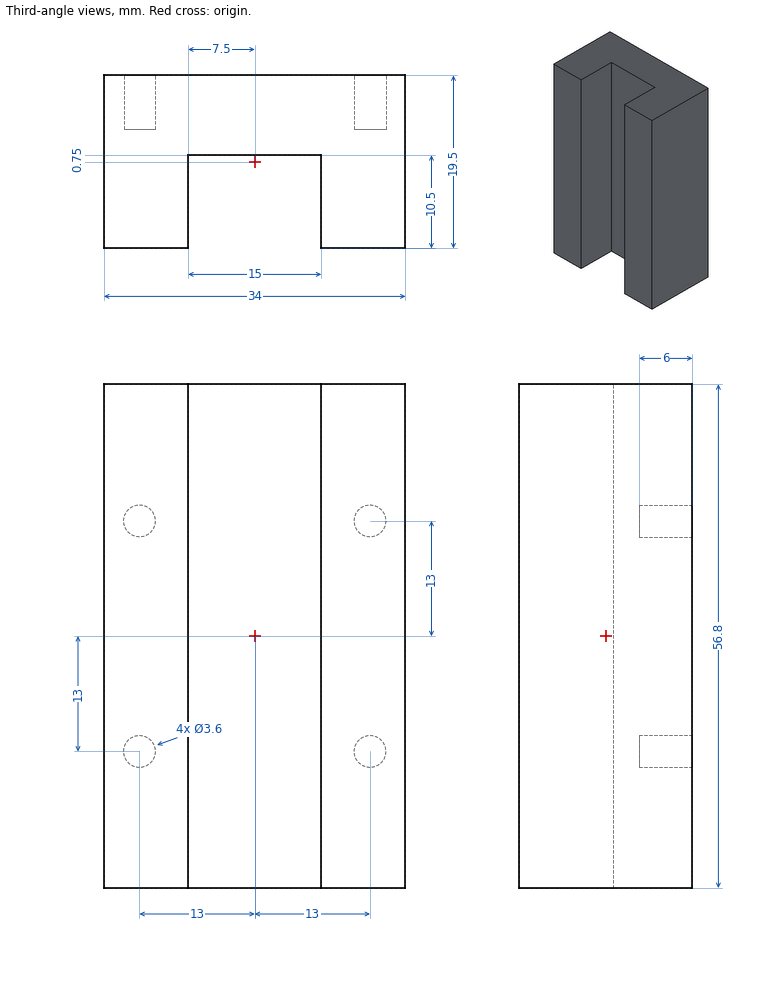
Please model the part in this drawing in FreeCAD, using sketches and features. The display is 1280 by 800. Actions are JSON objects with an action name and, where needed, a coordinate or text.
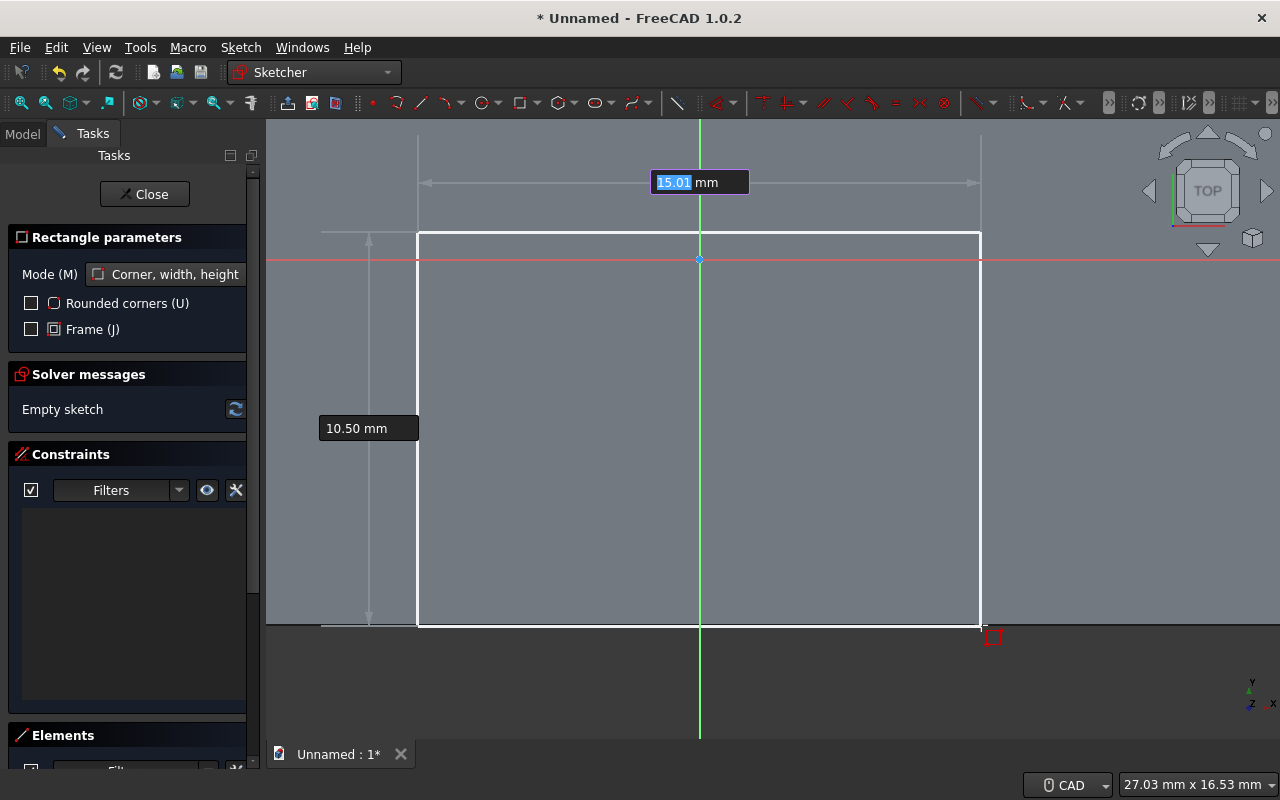
{"action": "type", "text": "15"}
{"action": "key", "text": "Tab"}
{"action": "type", "text": "10.5"}
{"action": "key", "text": "Return"}
{"action": "key", "text": "Escape"}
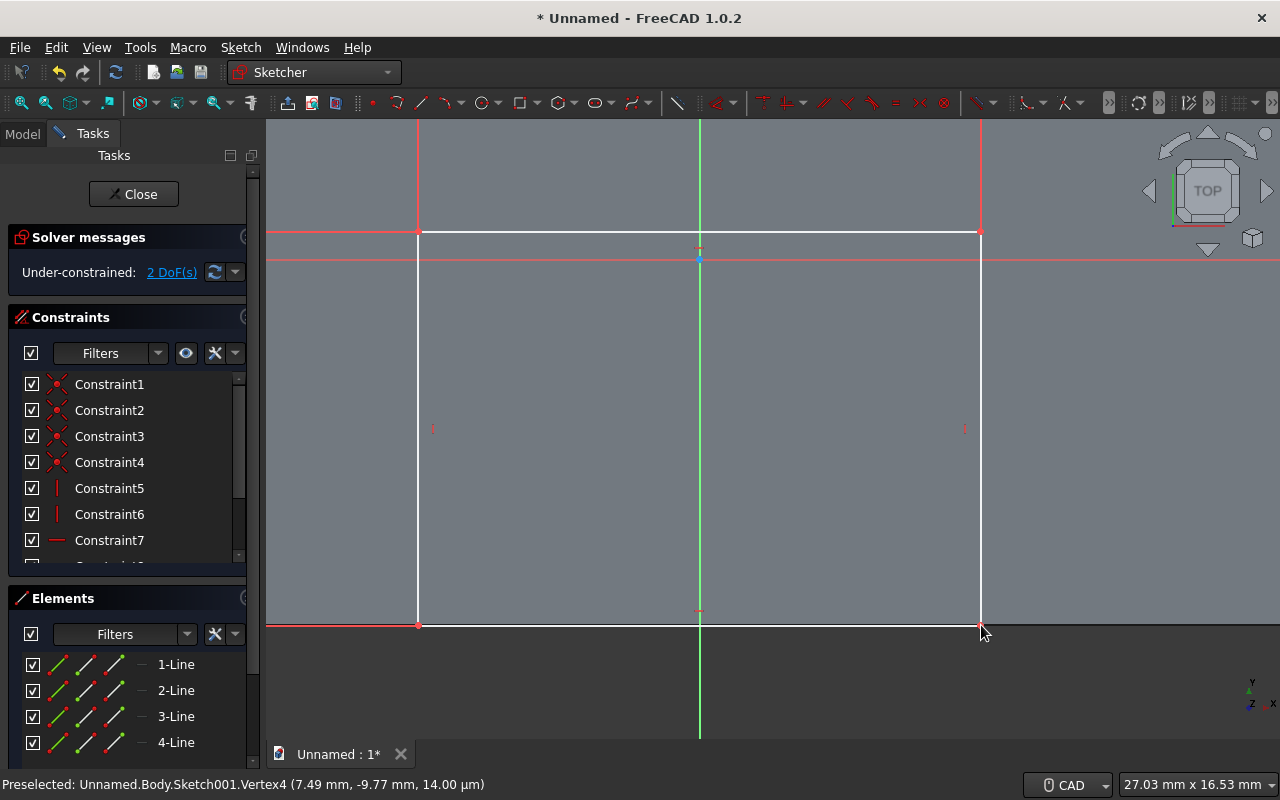
{"action": "left_click", "coordinate": [716, 104]}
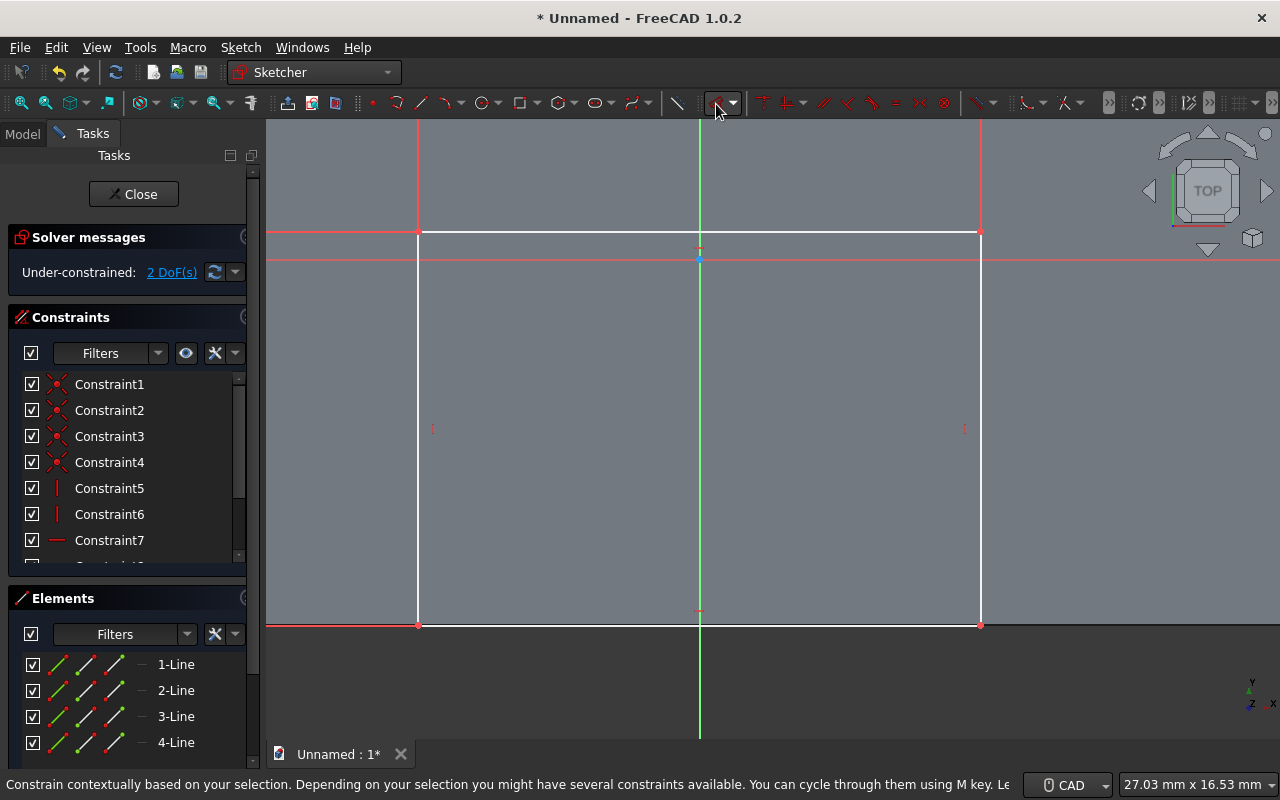
{"action": "left_click", "coordinate": [418, 232]}
{"action": "left_click", "coordinate": [559, 198]}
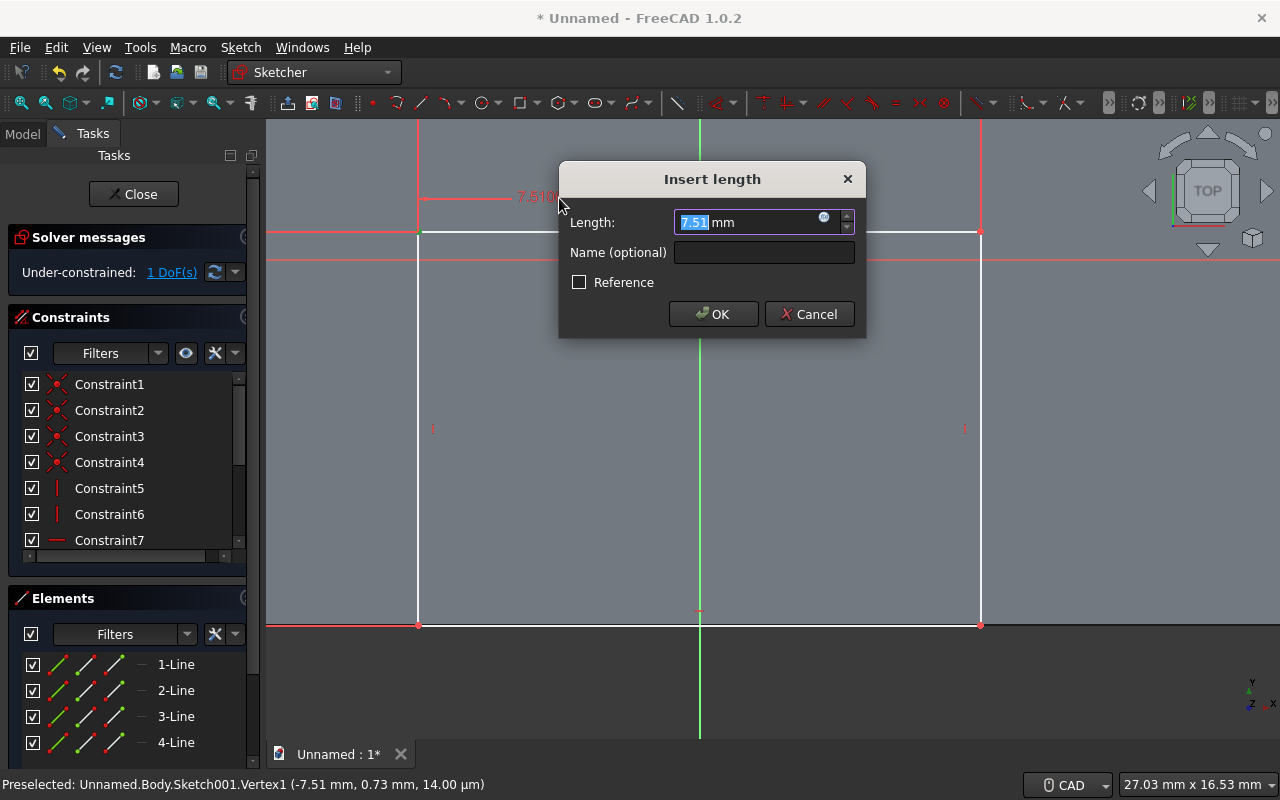
{"action": "type", "text": "7.5"}
{"action": "key", "text": "Return"}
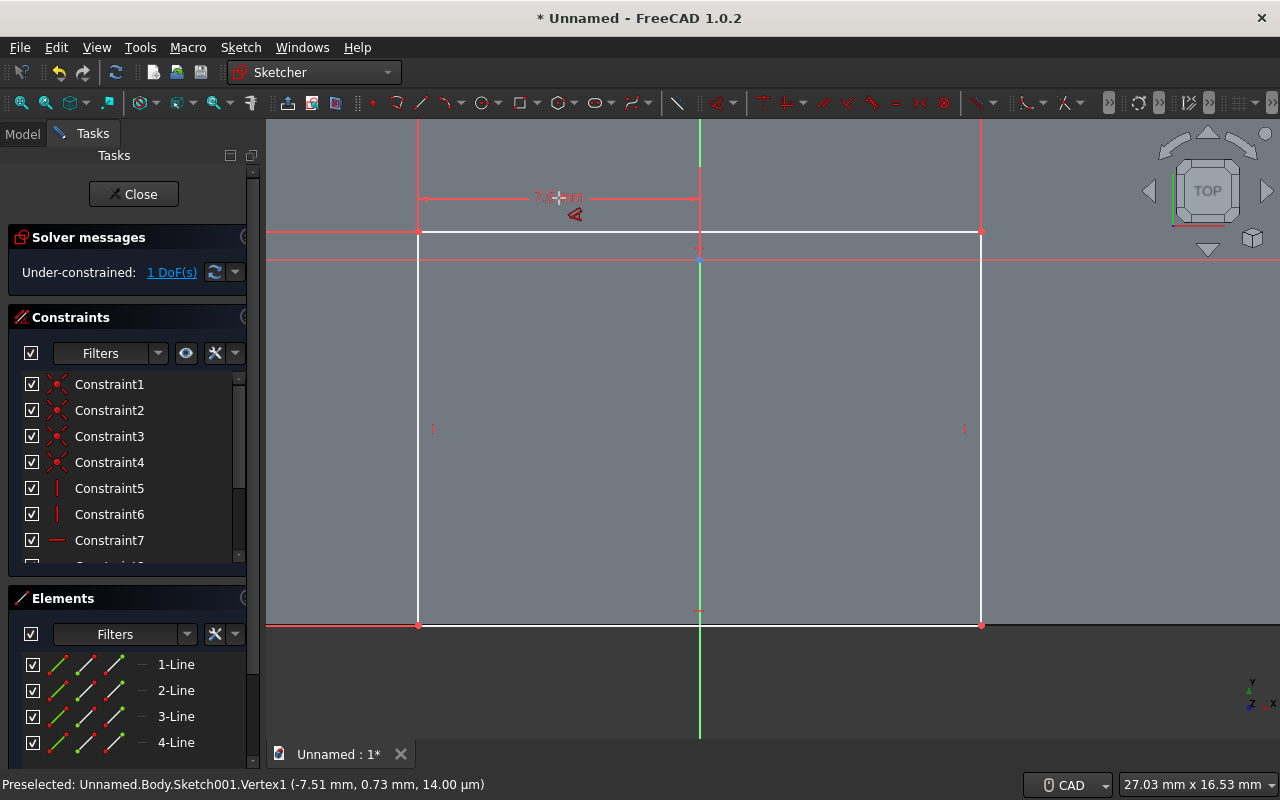
{"action": "scroll", "coordinate": [418, 232], "scroll_direction": "up", "scroll_amount": 2}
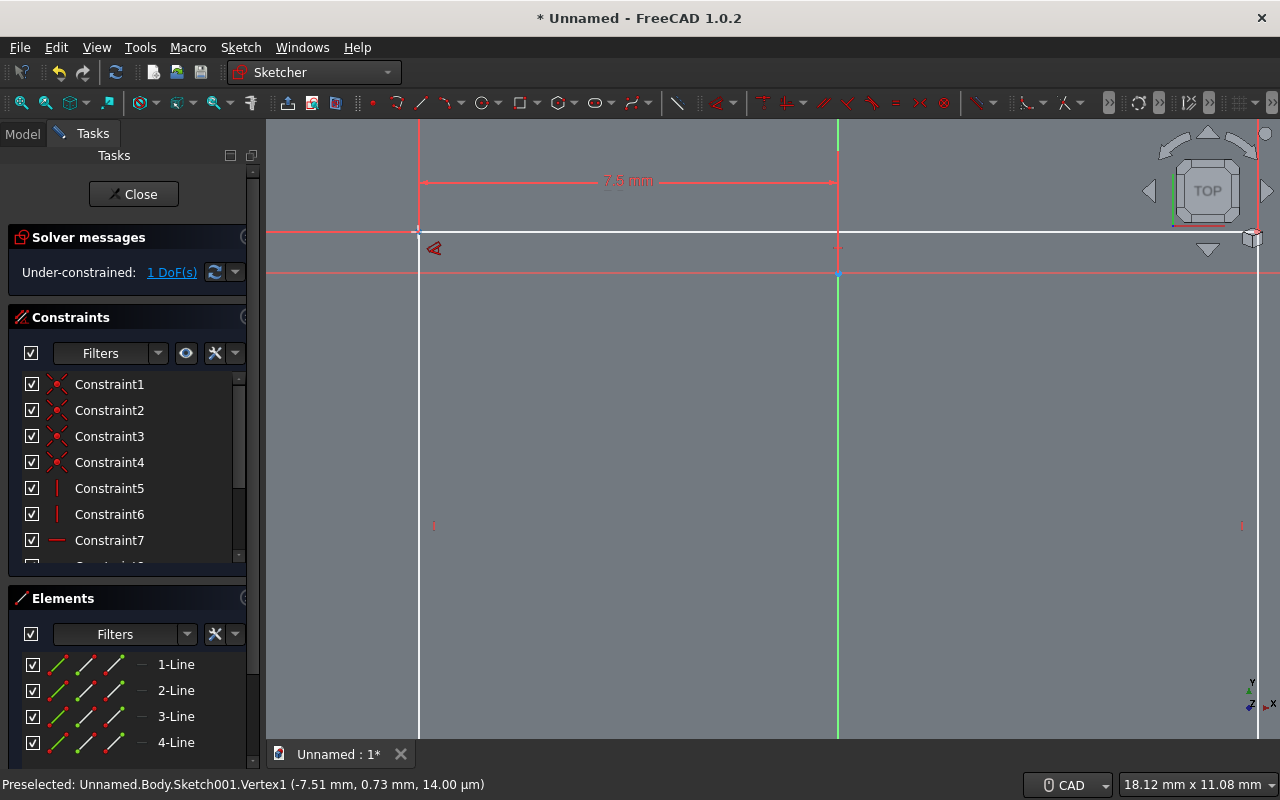
{"action": "left_click", "coordinate": [419, 232]}
{"action": "left_click", "coordinate": [385, 252]}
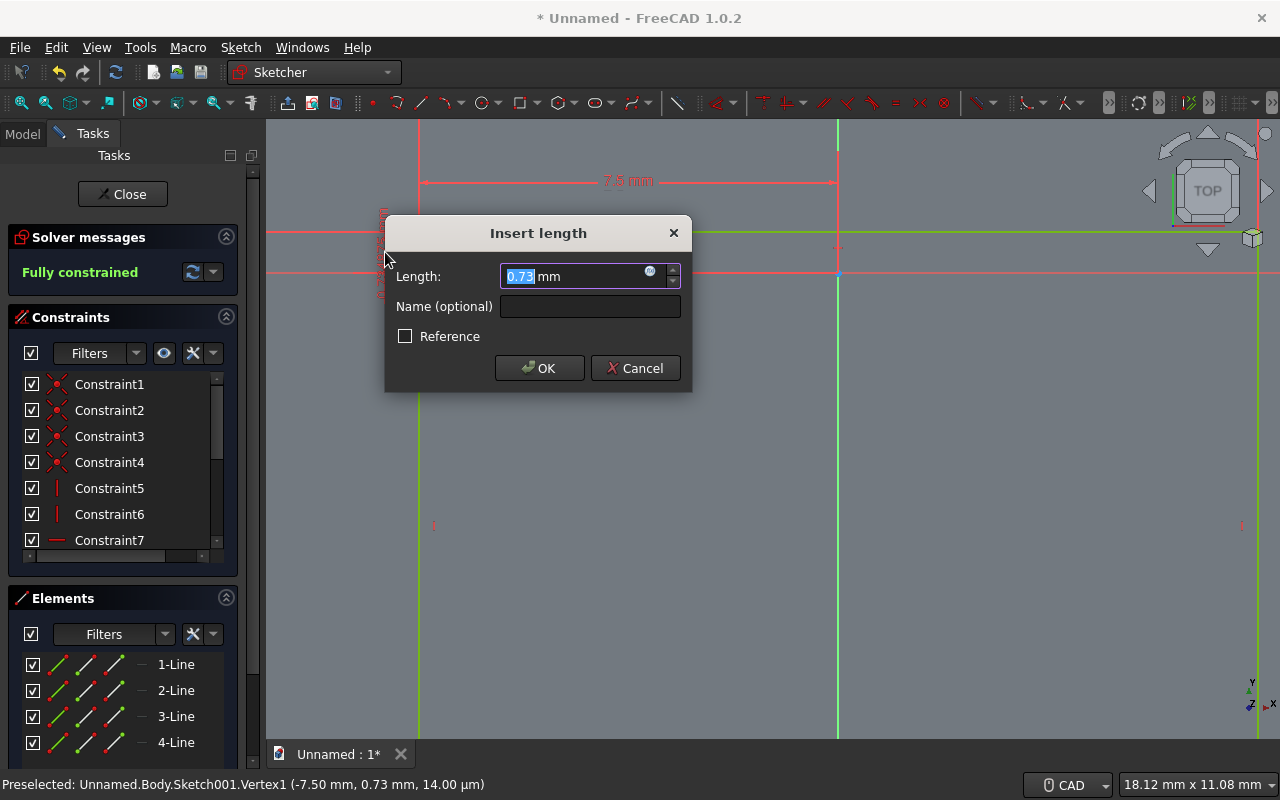
{"action": "type", "text": "0.75"}
{"action": "key", "text": "Return"}
{"action": "key", "text": "Escape"}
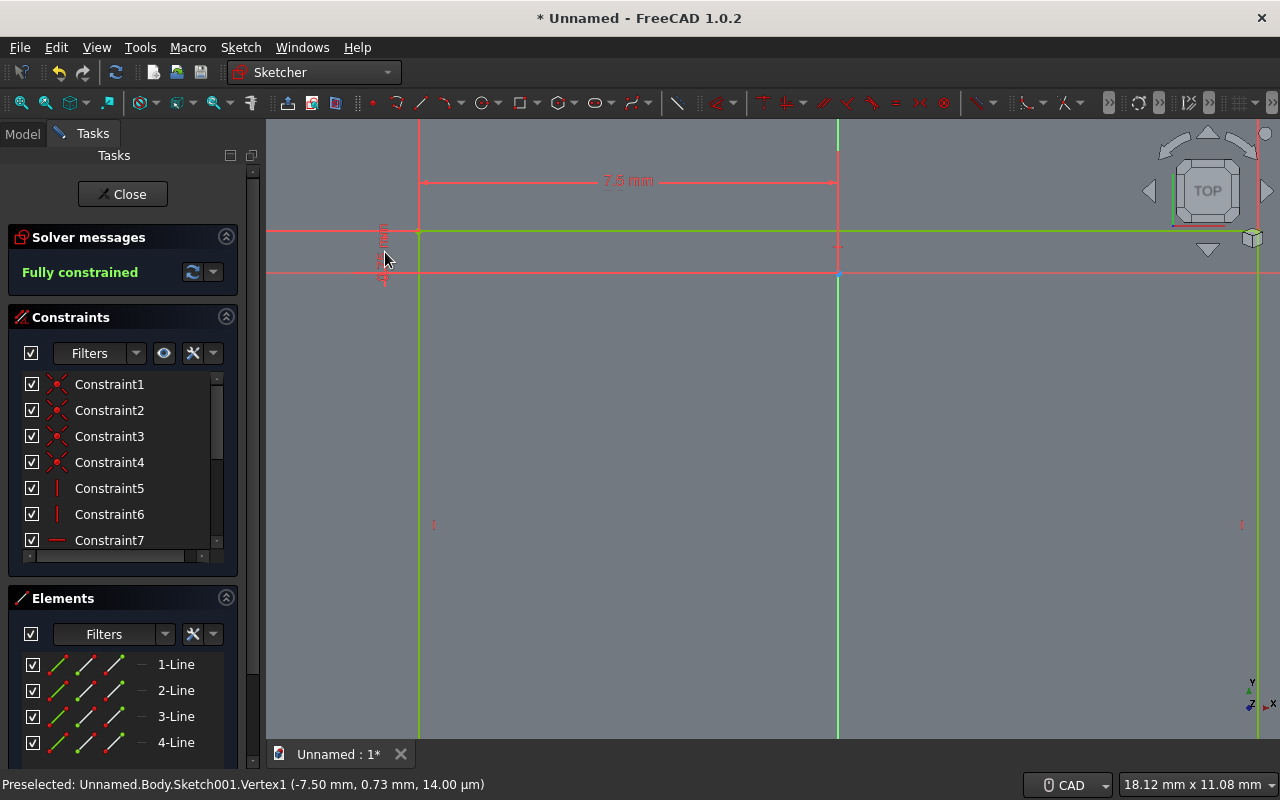
{"action": "left_click", "coordinate": [123, 194]}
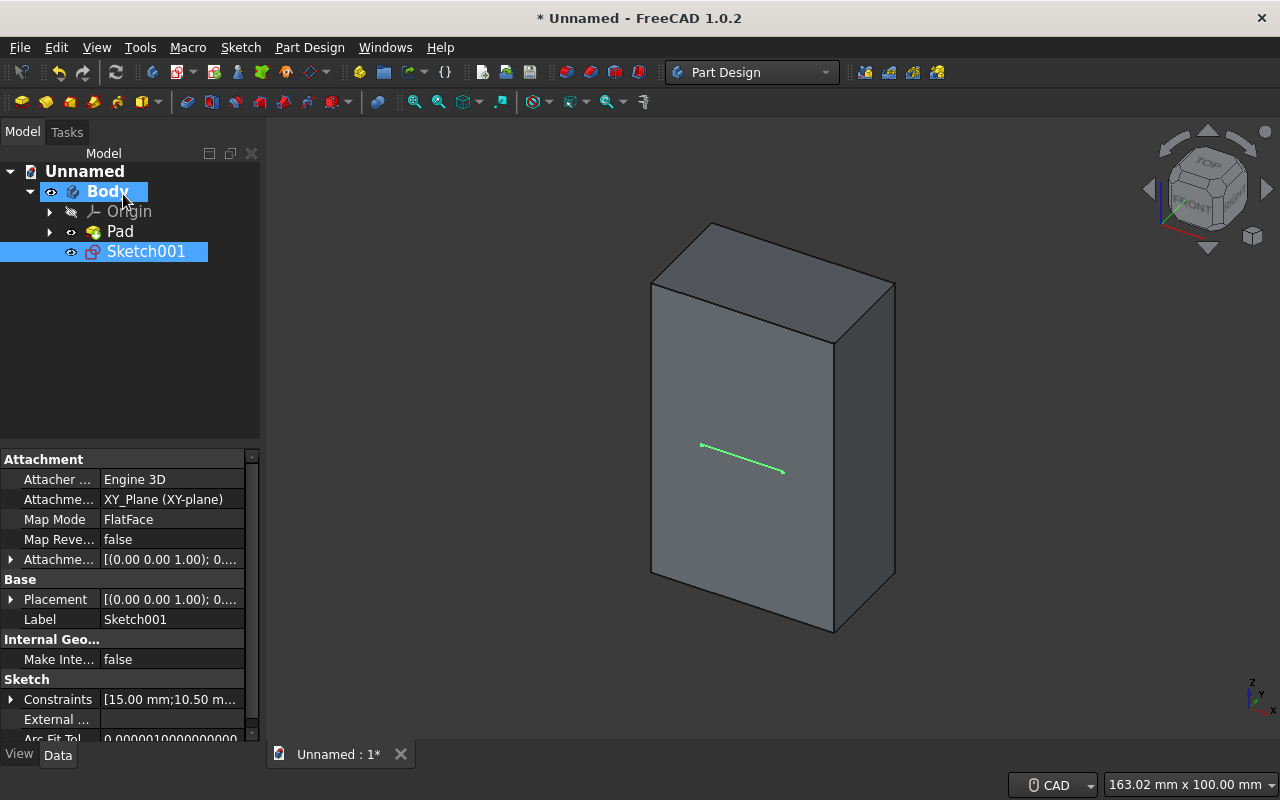
{"action": "left_click", "coordinate": [188, 102]}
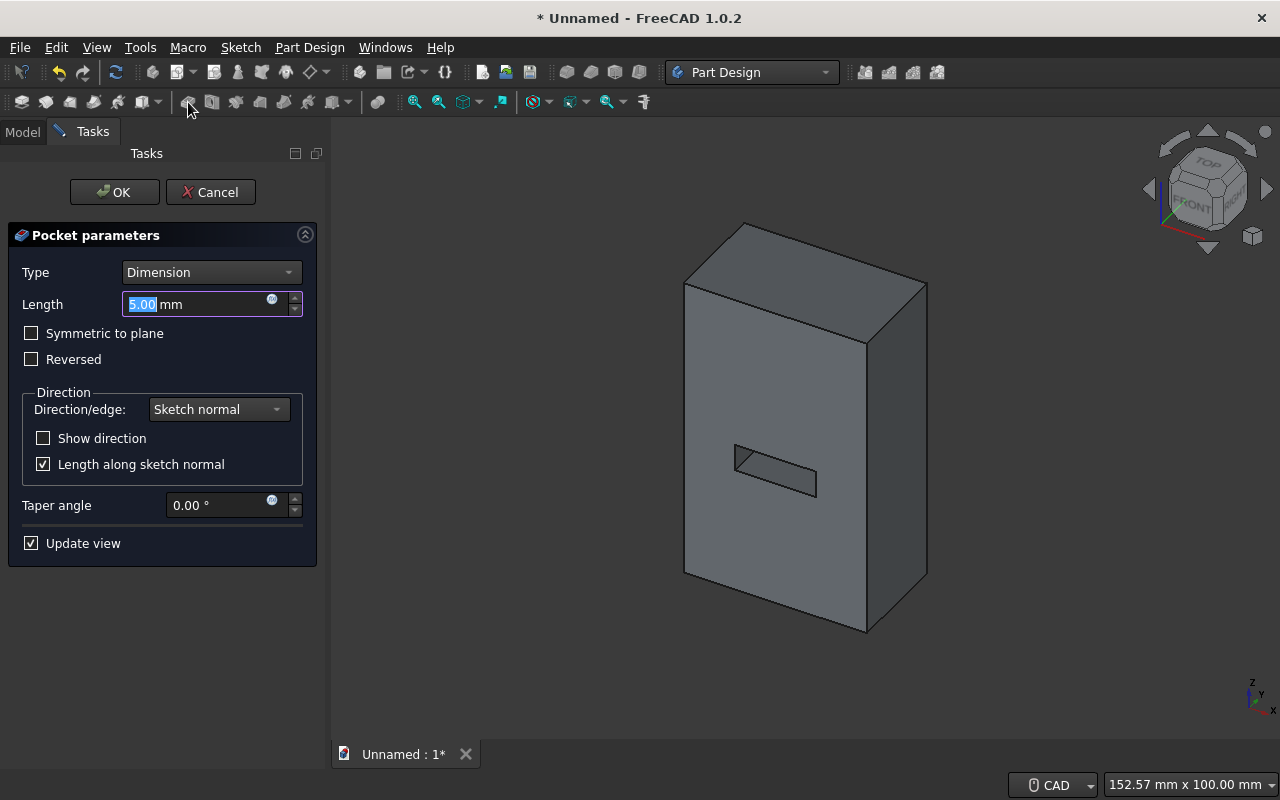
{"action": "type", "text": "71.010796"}
{"action": "key", "text": "Tab"}